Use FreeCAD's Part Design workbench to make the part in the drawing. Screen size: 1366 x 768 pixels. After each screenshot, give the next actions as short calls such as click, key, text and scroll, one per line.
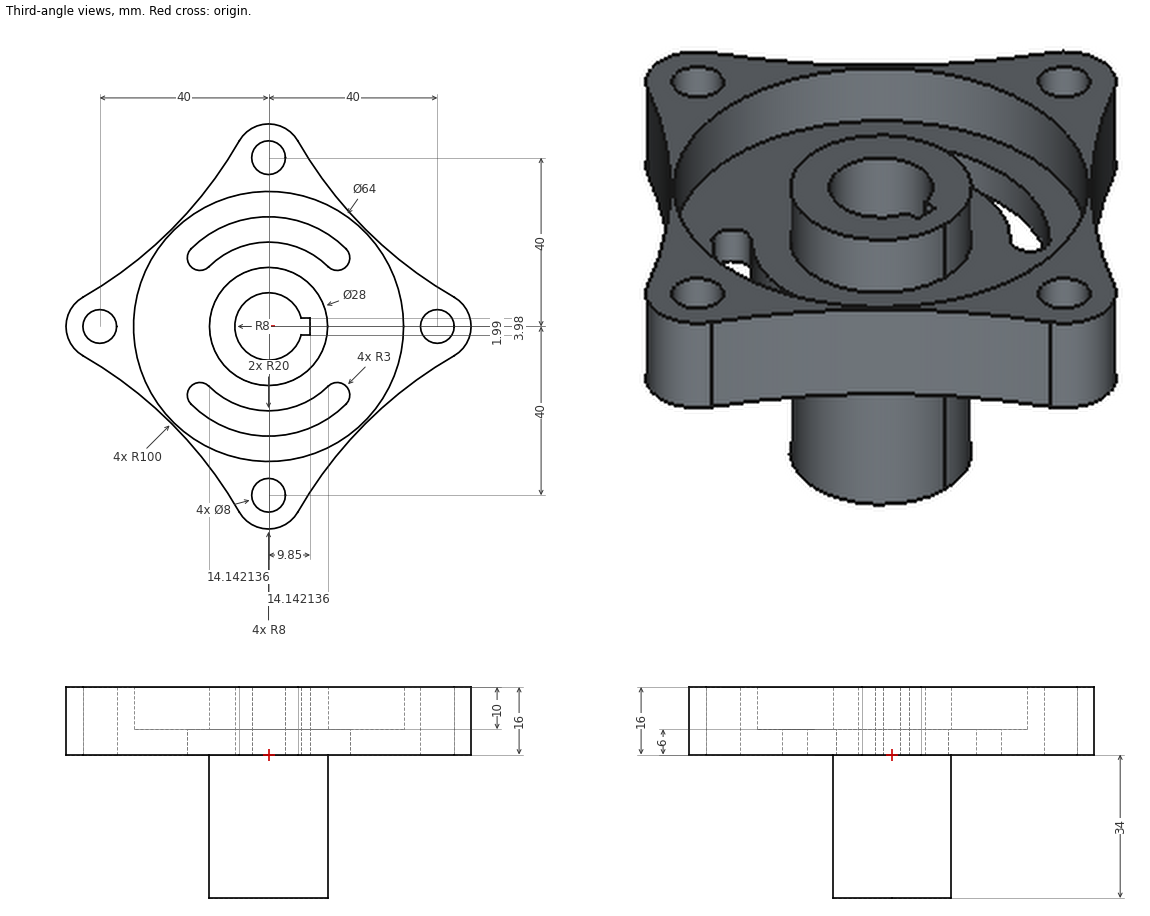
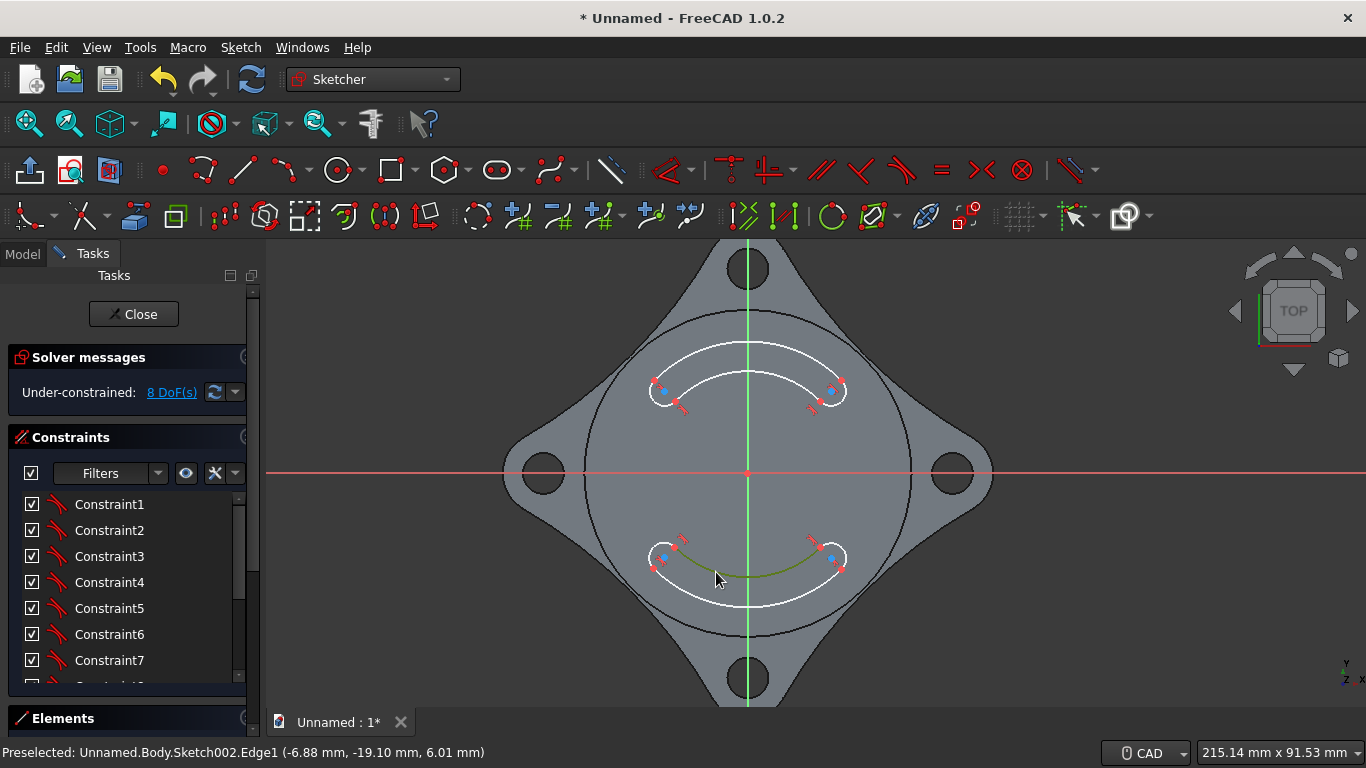
click(780, 376)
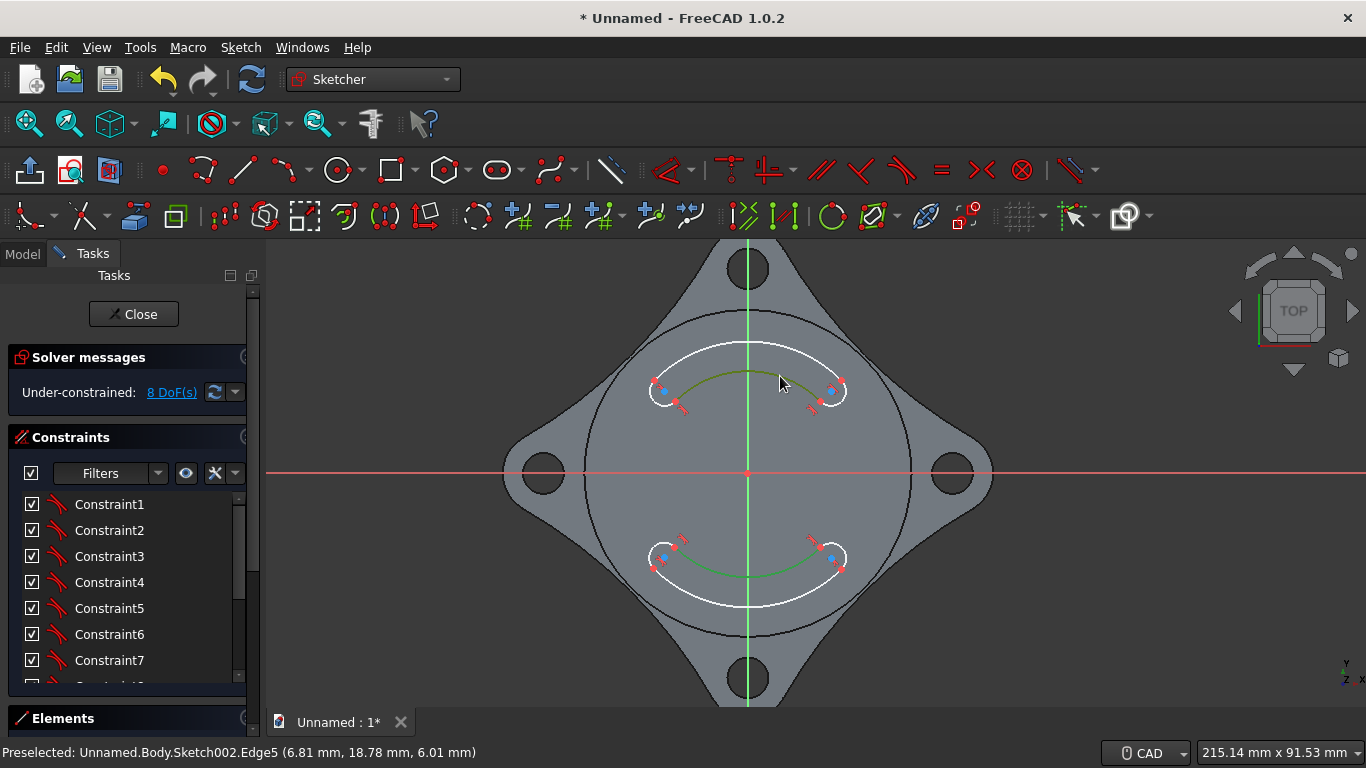
click(942, 170)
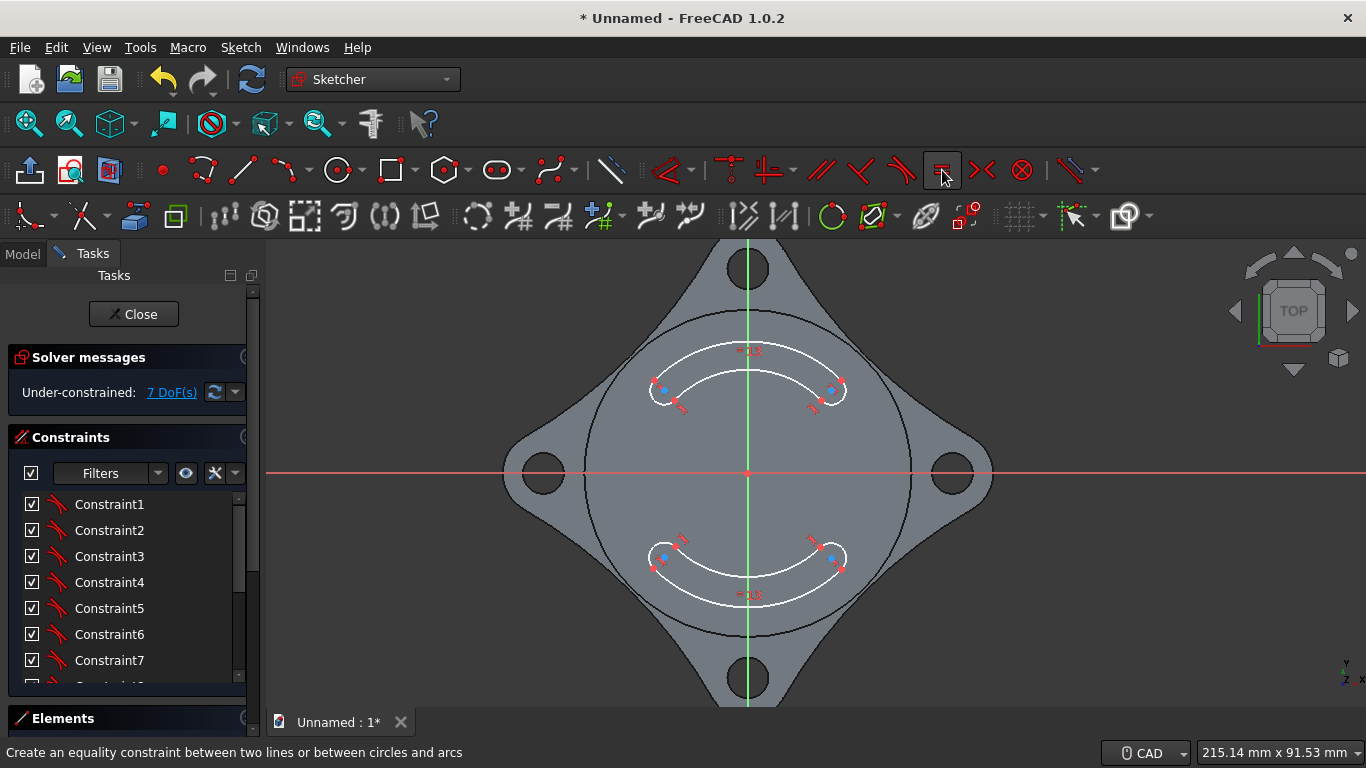
click(662, 543)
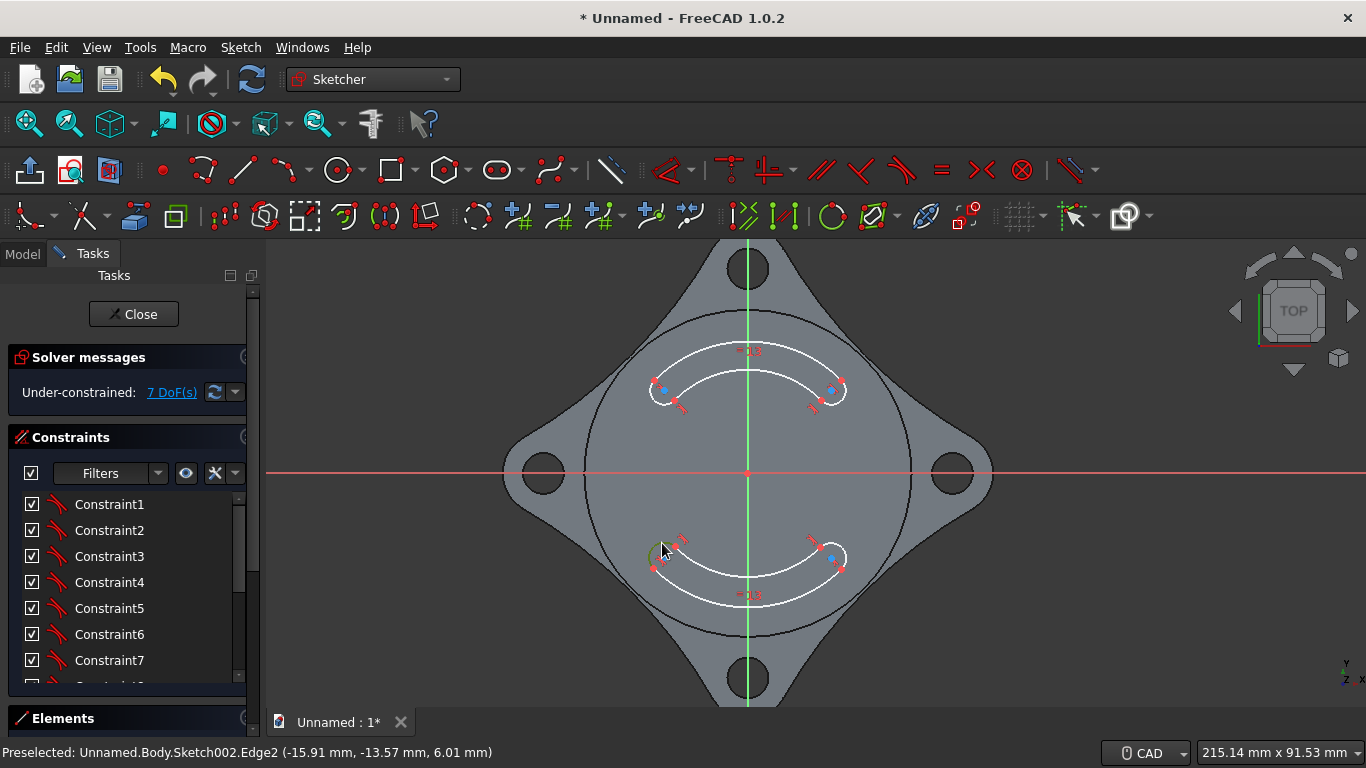
click(834, 405)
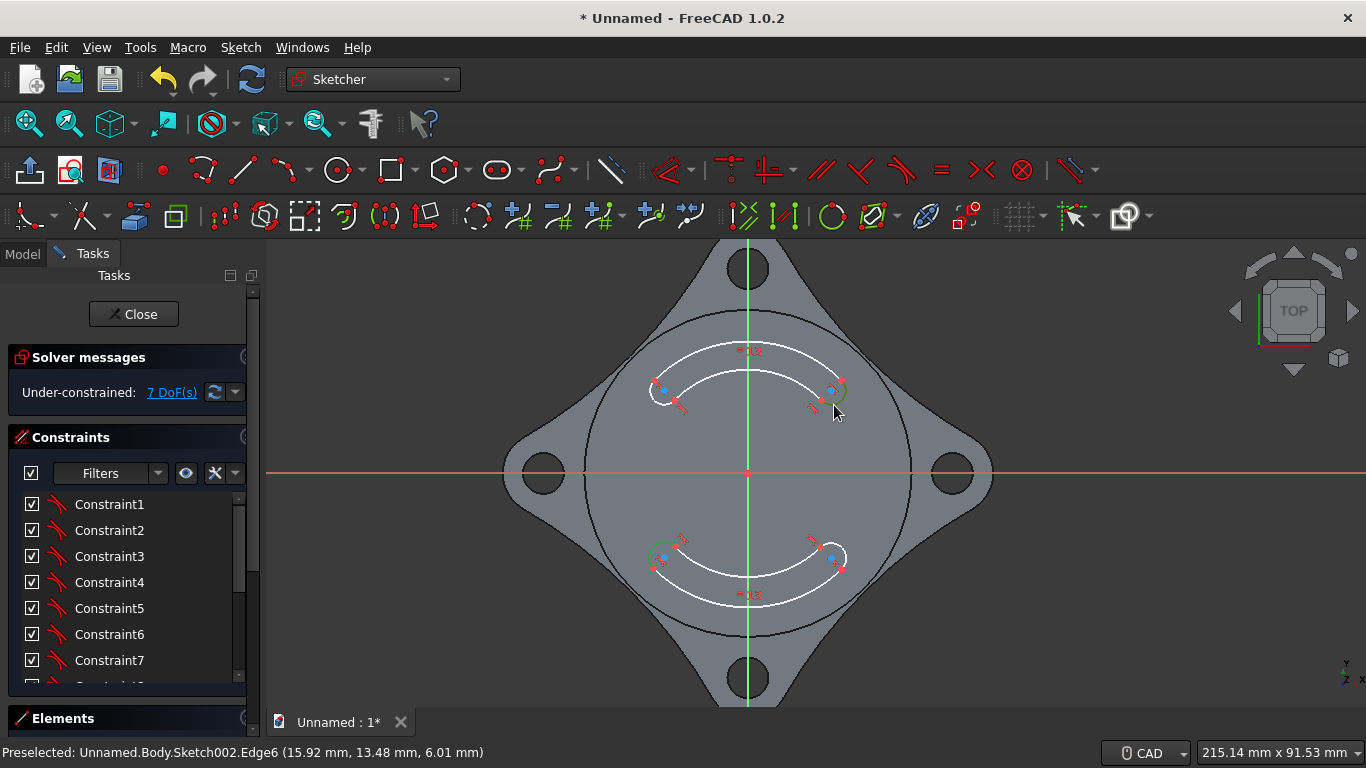
click(942, 170)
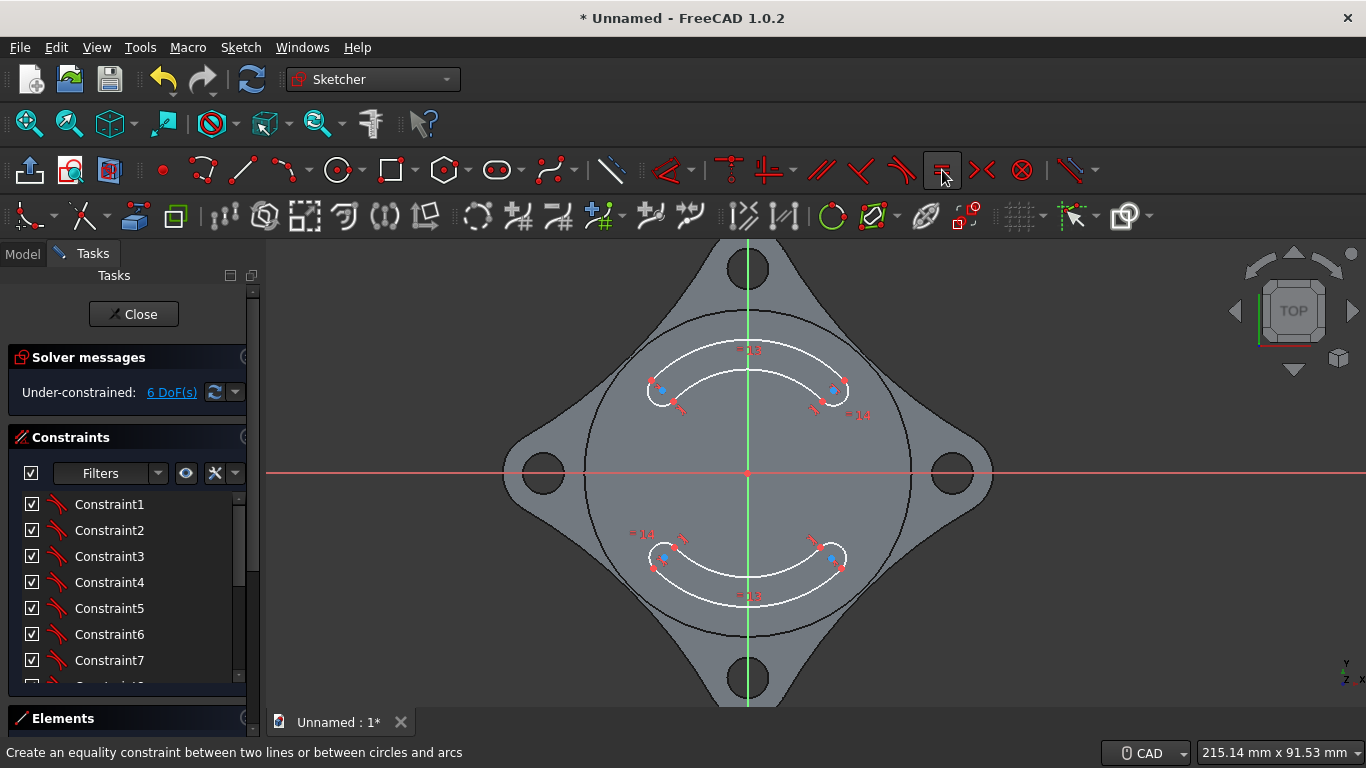
key(d)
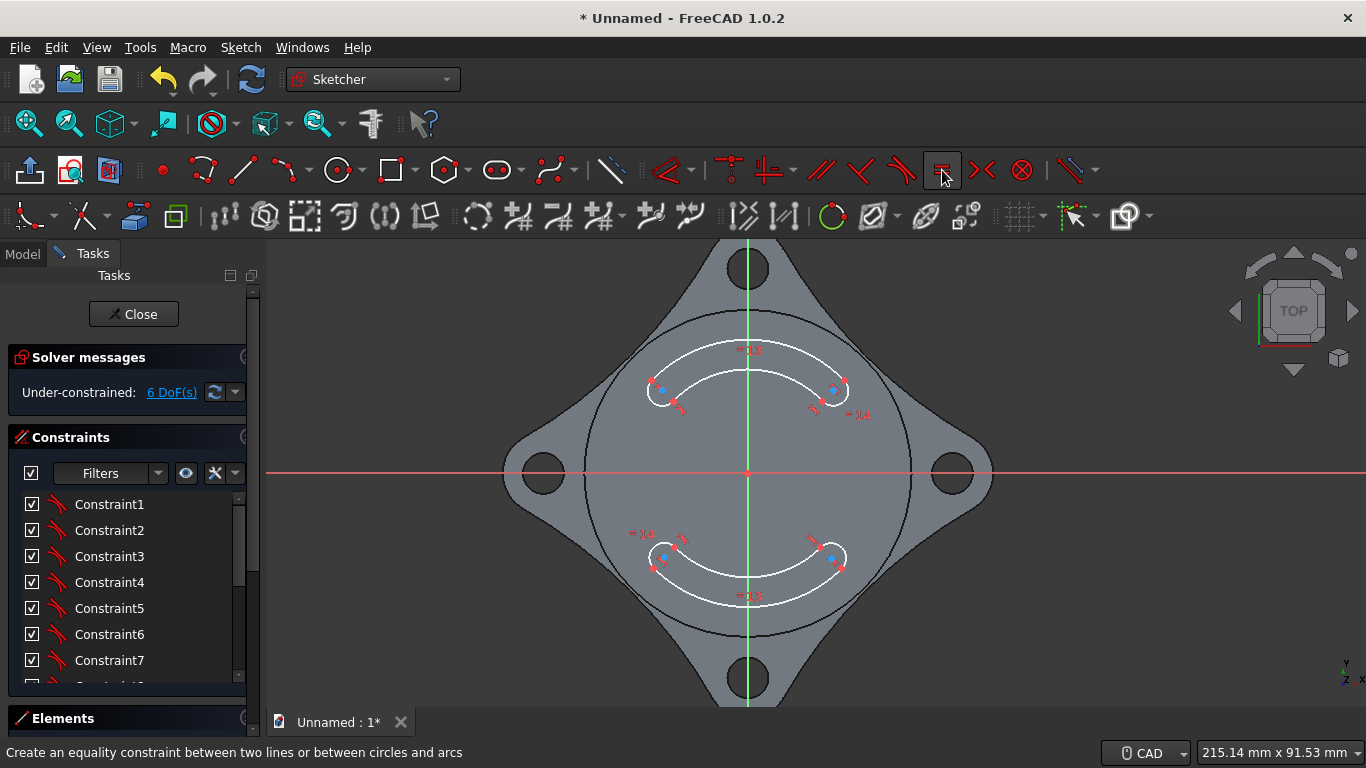
click(716, 572)
click(617, 508)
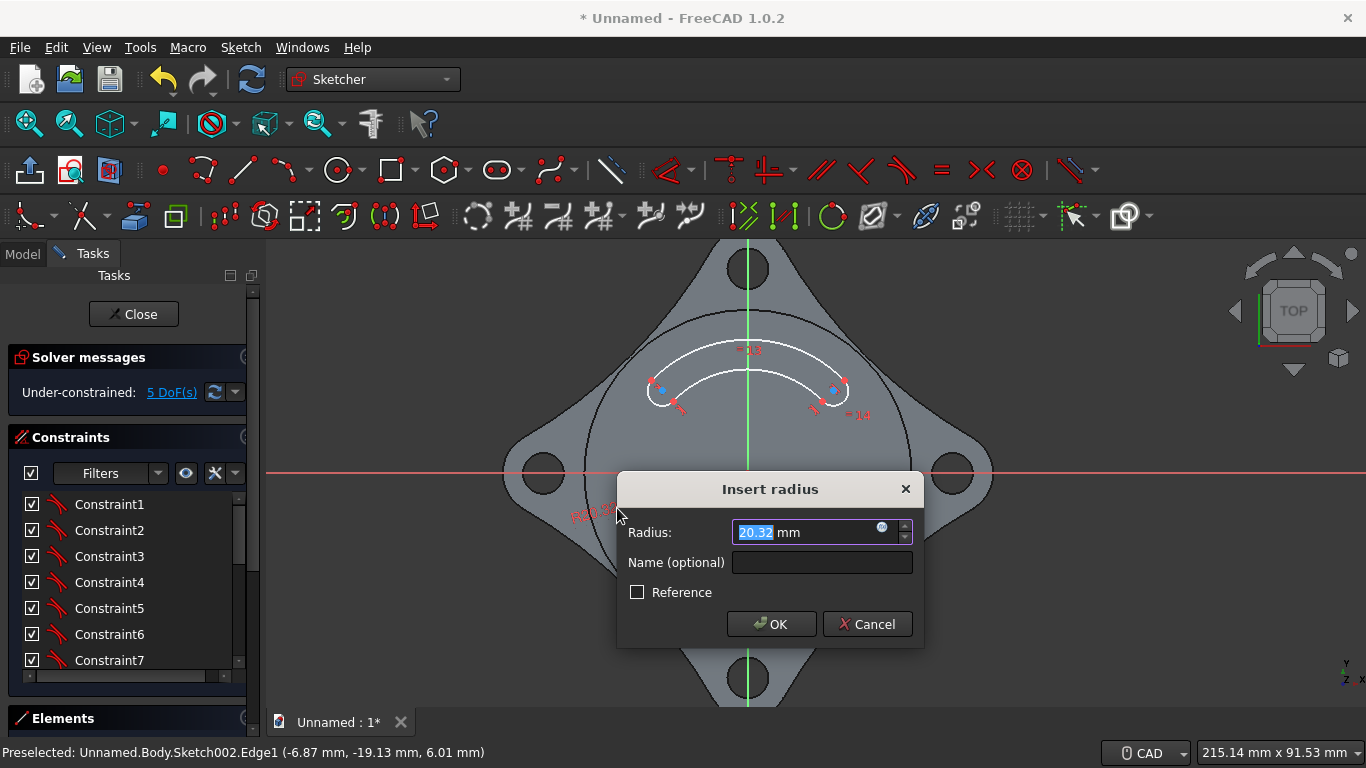
text(20)
key(Return)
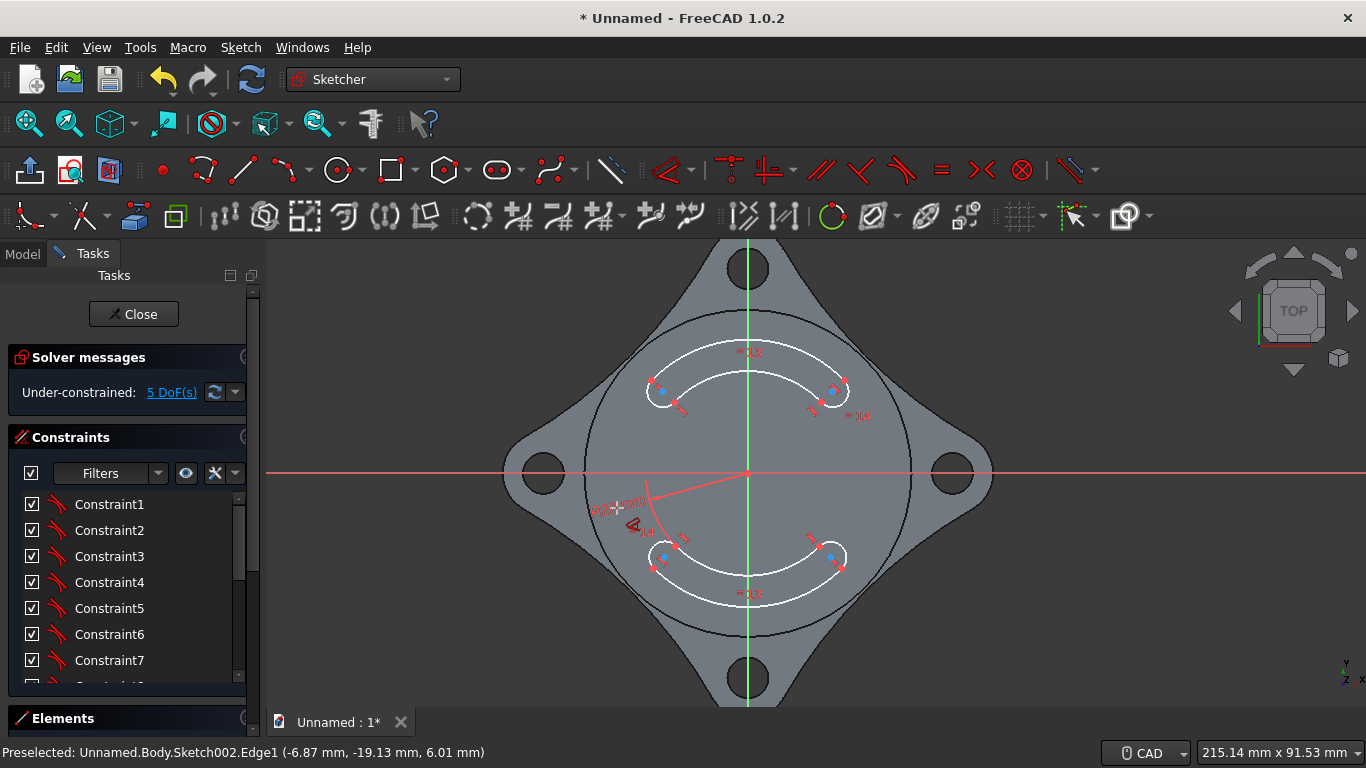
scroll(662, 542, up, 5)